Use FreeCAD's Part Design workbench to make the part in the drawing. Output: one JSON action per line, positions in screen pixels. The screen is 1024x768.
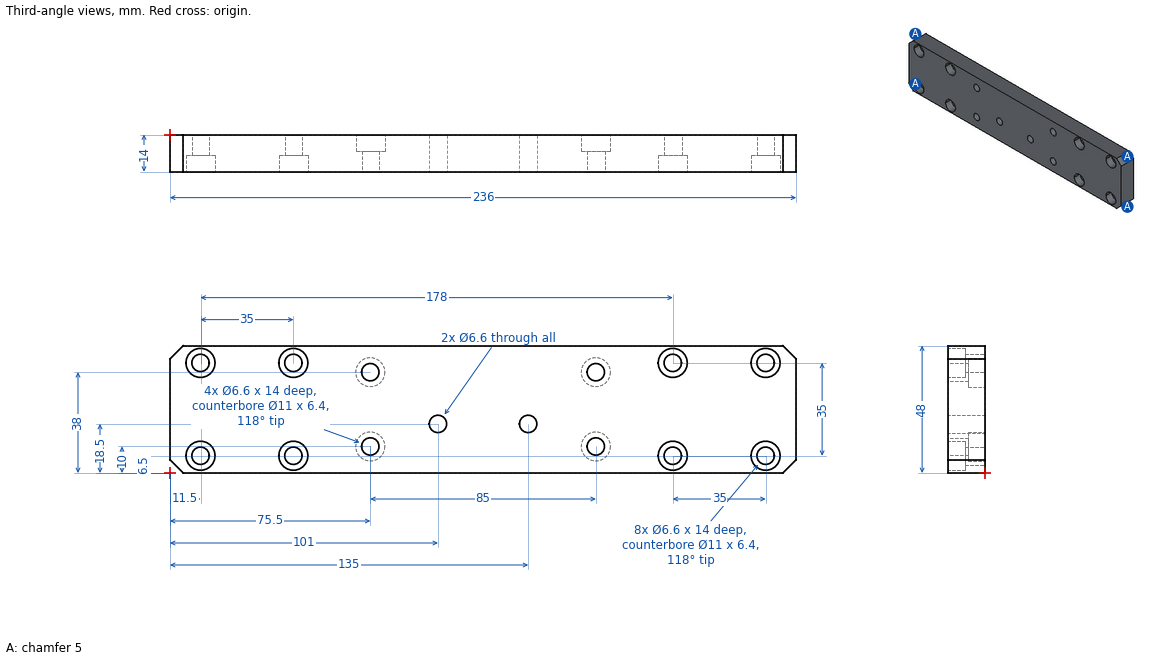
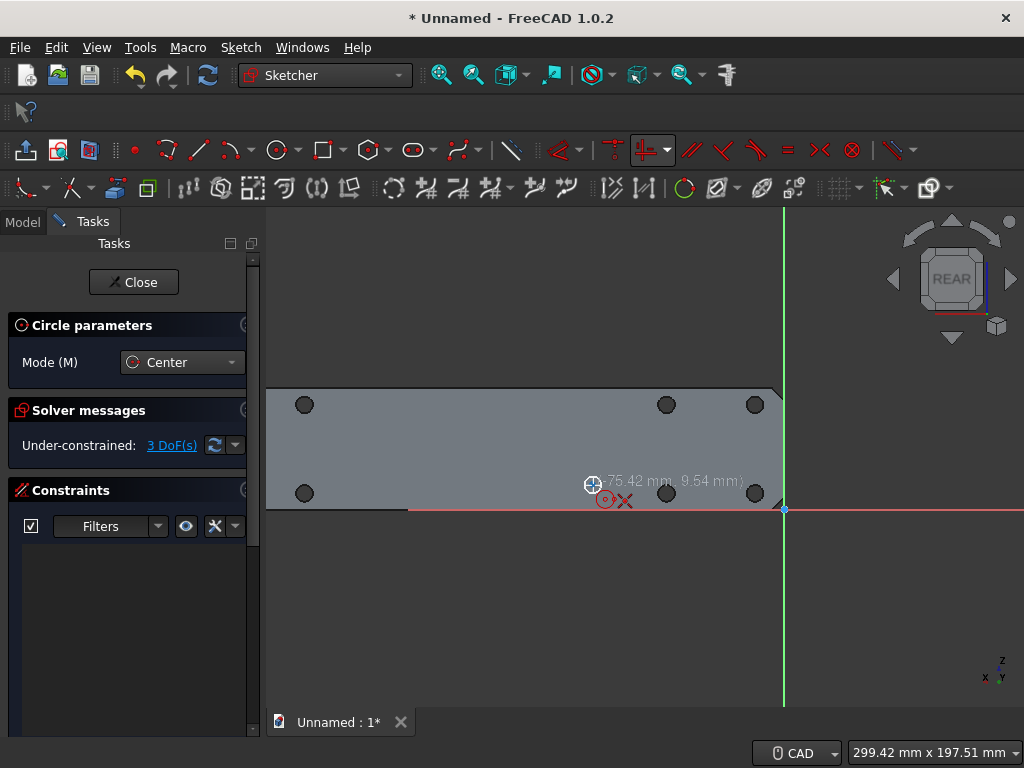
{"action": "scroll", "coordinate": [378, 485], "scroll_direction": "up", "scroll_amount": 5}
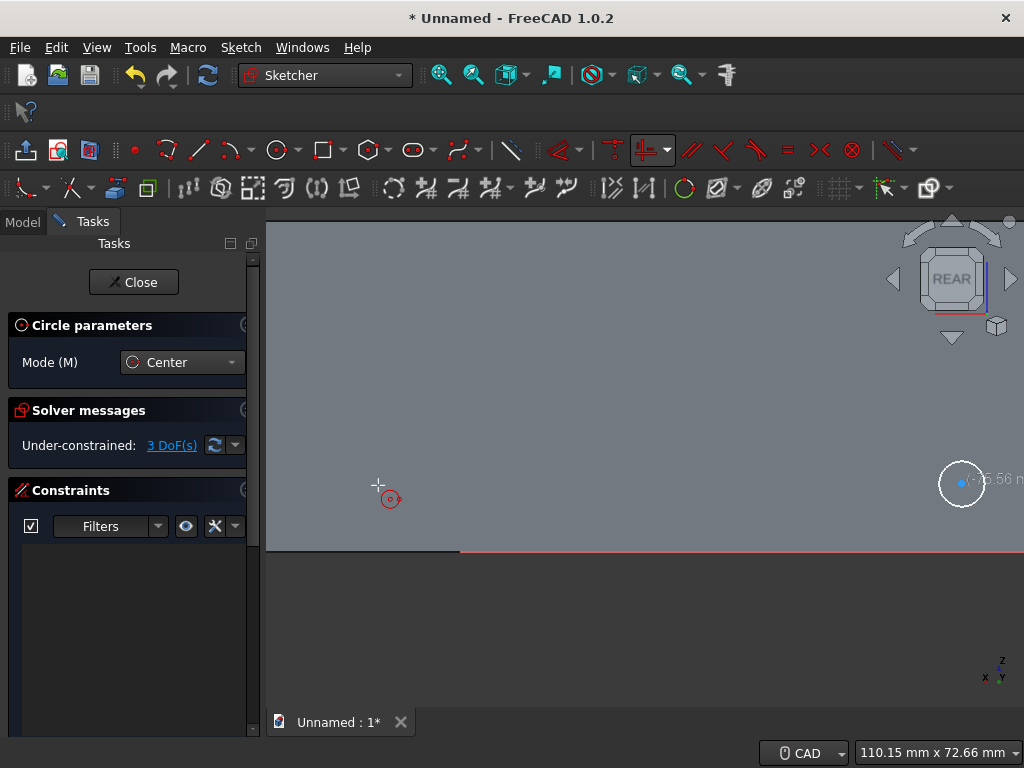
{"action": "left_click", "coordinate": [377, 483]}
{"action": "left_click", "coordinate": [393, 467]}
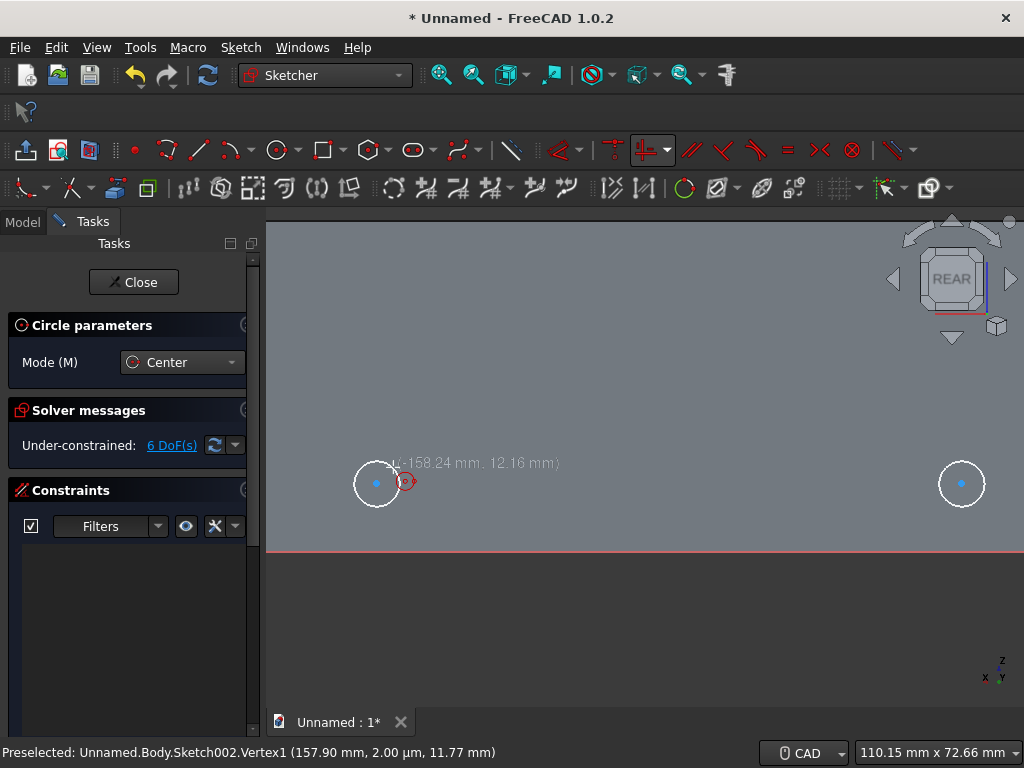
{"action": "scroll", "coordinate": [378, 485], "scroll_direction": "down", "scroll_amount": 5}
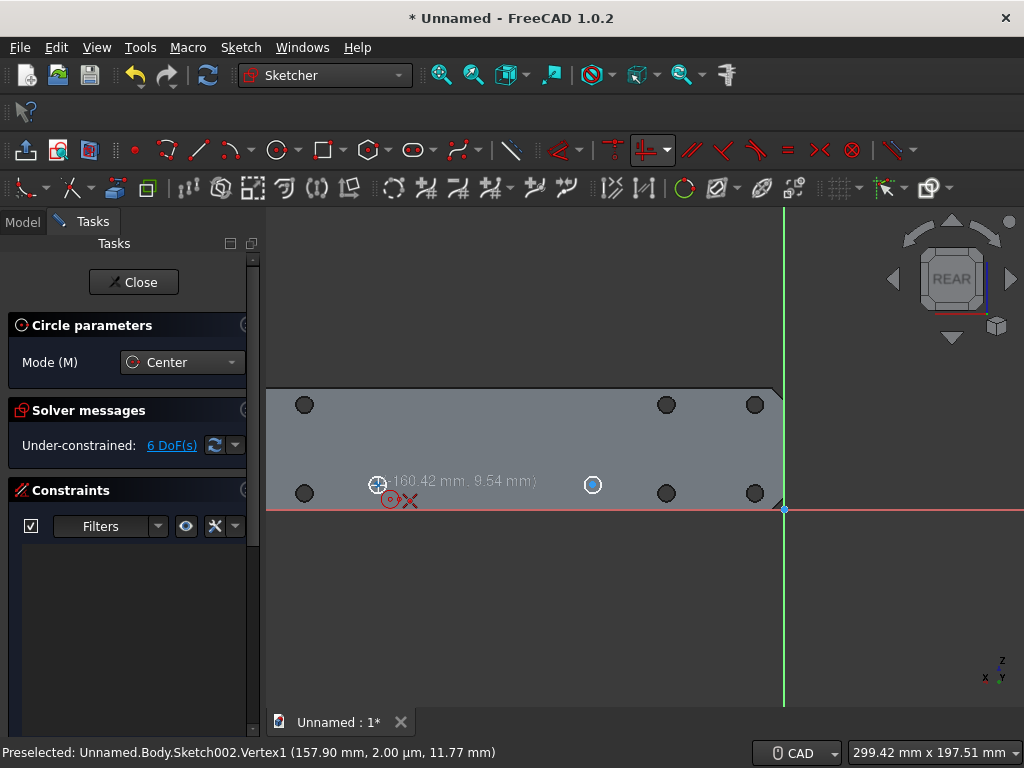
{"action": "scroll", "coordinate": [593, 414], "scroll_direction": "up", "scroll_amount": 5}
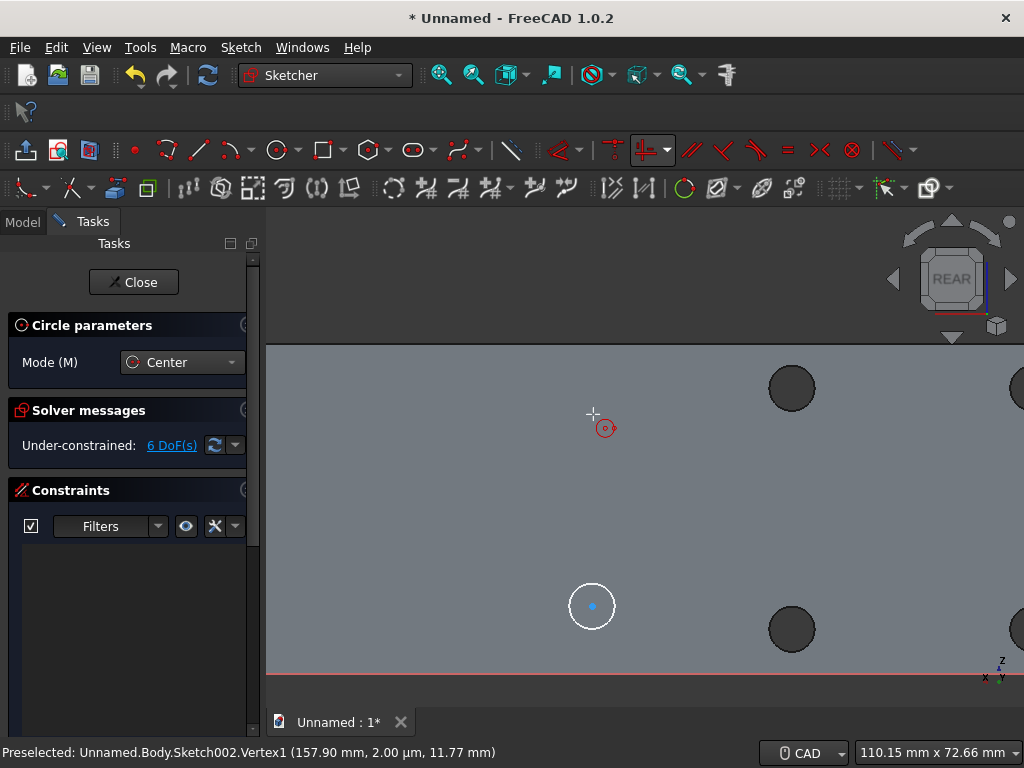
{"action": "left_click", "coordinate": [592, 412]}
{"action": "left_click", "coordinate": [608, 396]}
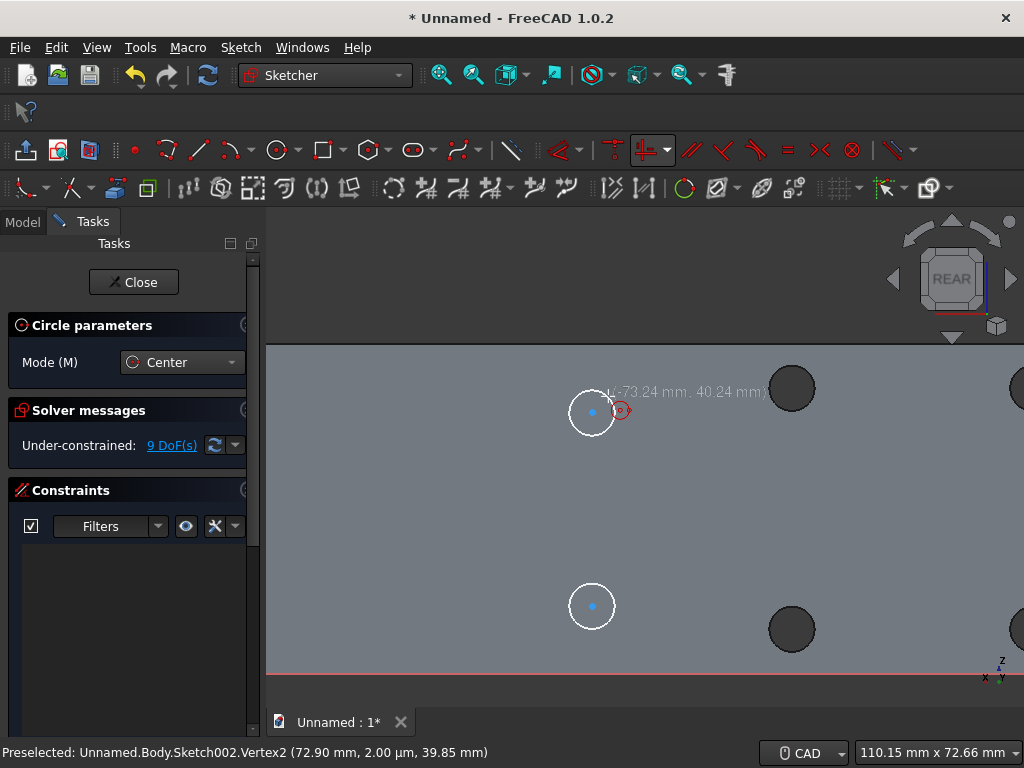
{"action": "scroll", "coordinate": [593, 413], "scroll_direction": "down", "scroll_amount": 5}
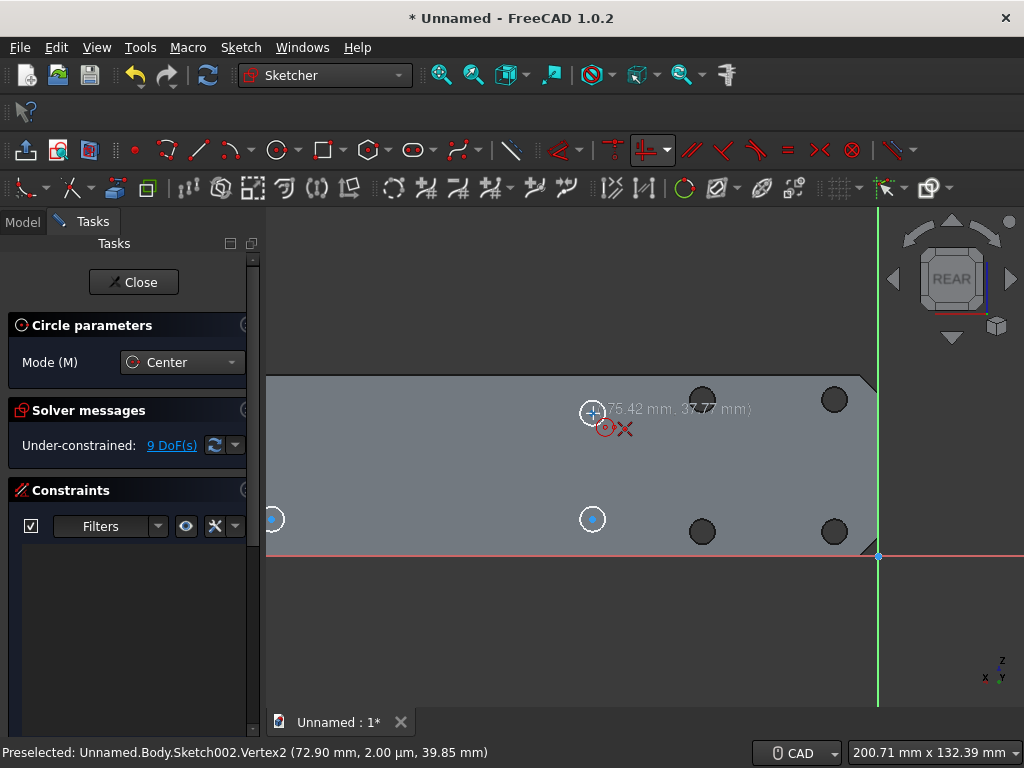
{"action": "scroll", "coordinate": [378, 413], "scroll_direction": "up", "scroll_amount": 5}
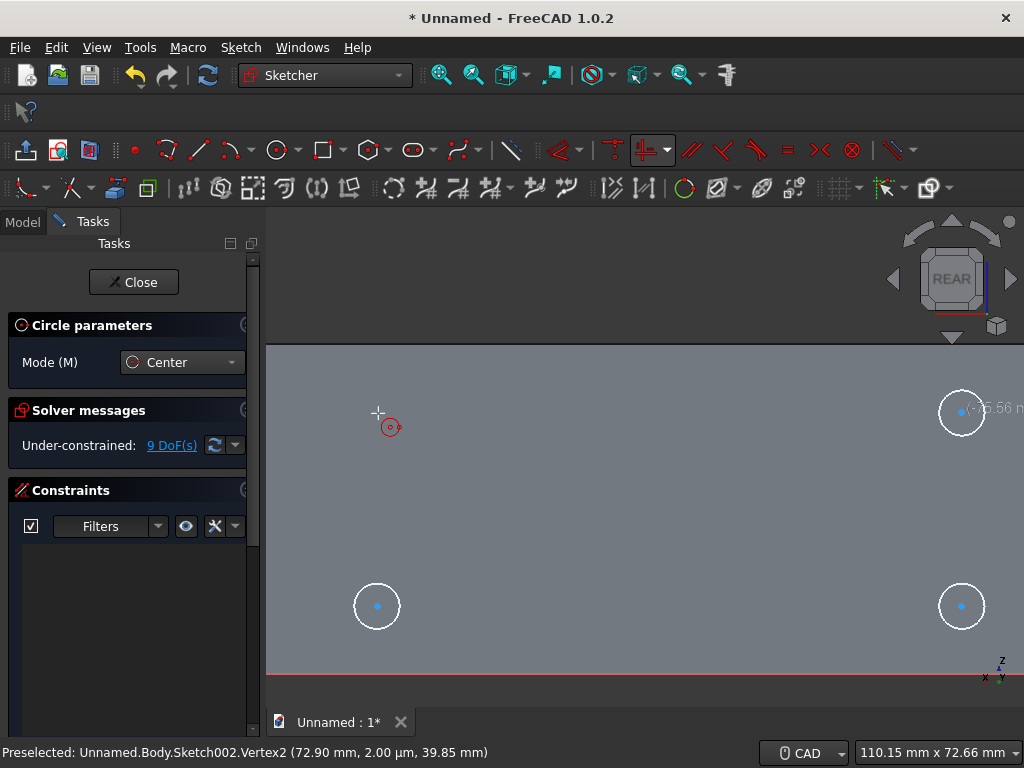
{"action": "left_click", "coordinate": [377, 412]}
{"action": "left_click", "coordinate": [393, 396]}
{"action": "key", "text": "Escape"}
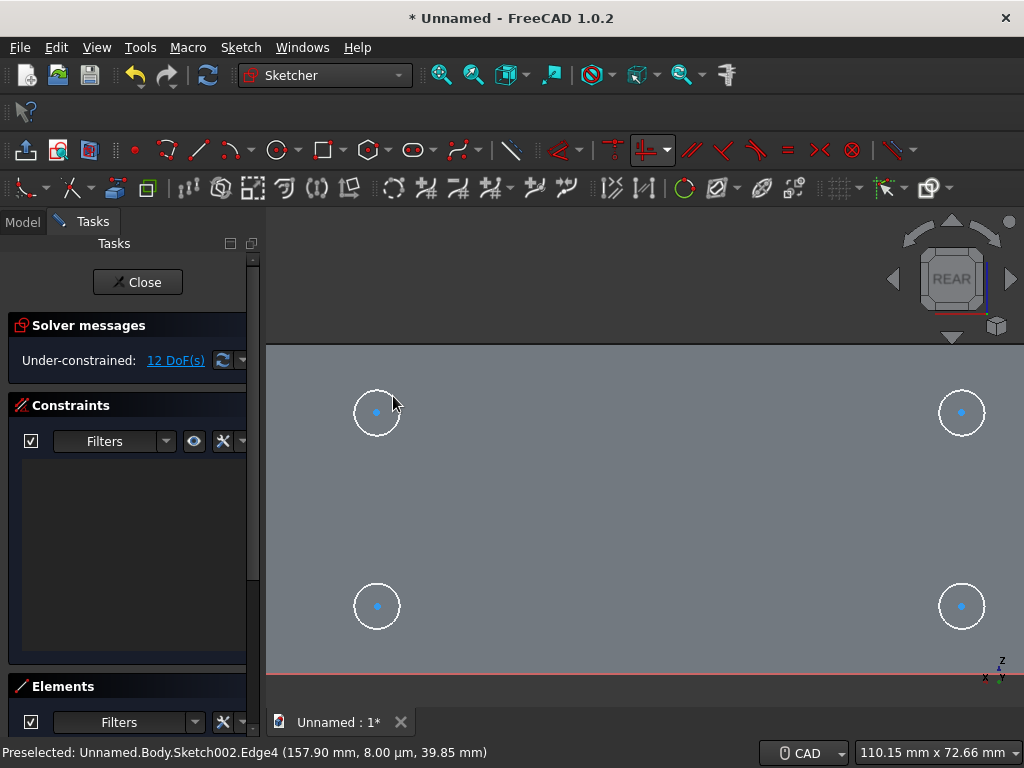
{"action": "scroll", "coordinate": [378, 413], "scroll_direction": "down", "scroll_amount": 5}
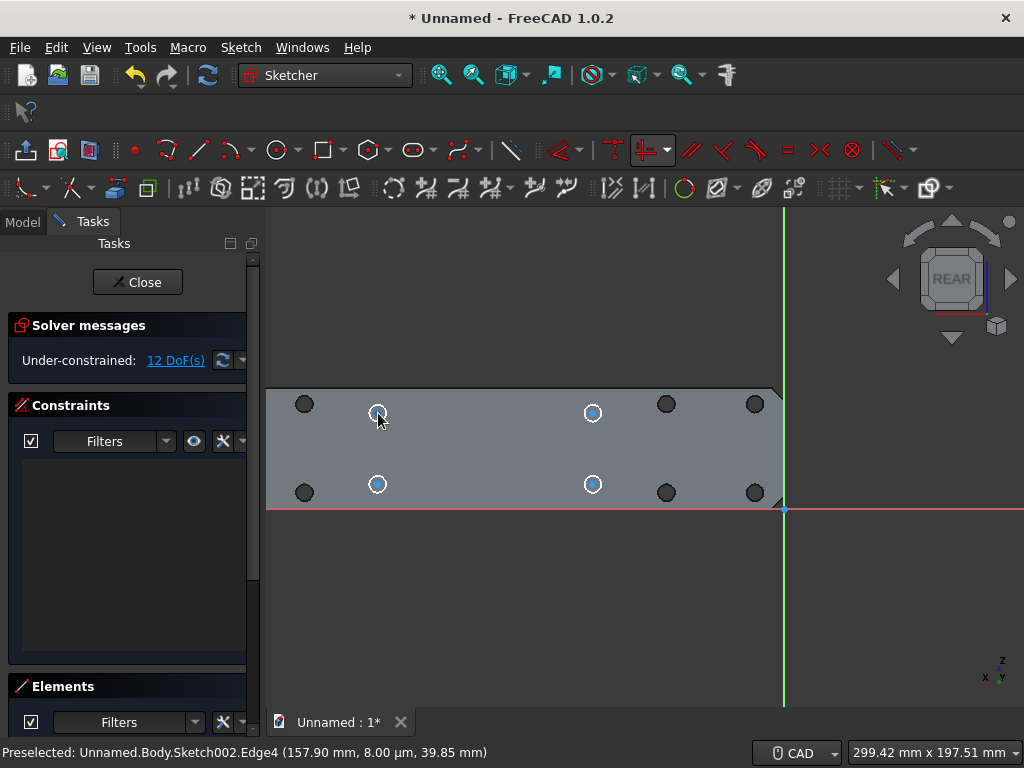
{"action": "scroll", "coordinate": [599, 478], "scroll_direction": "up", "scroll_amount": 3}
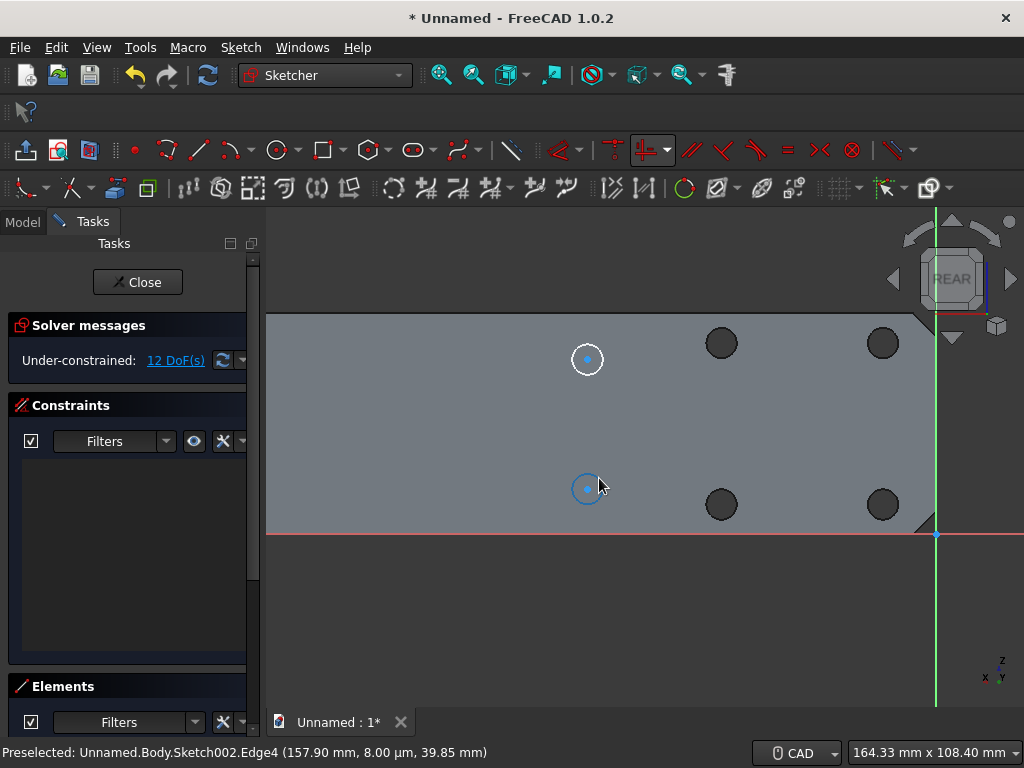
{"action": "left_click", "coordinate": [598, 478]}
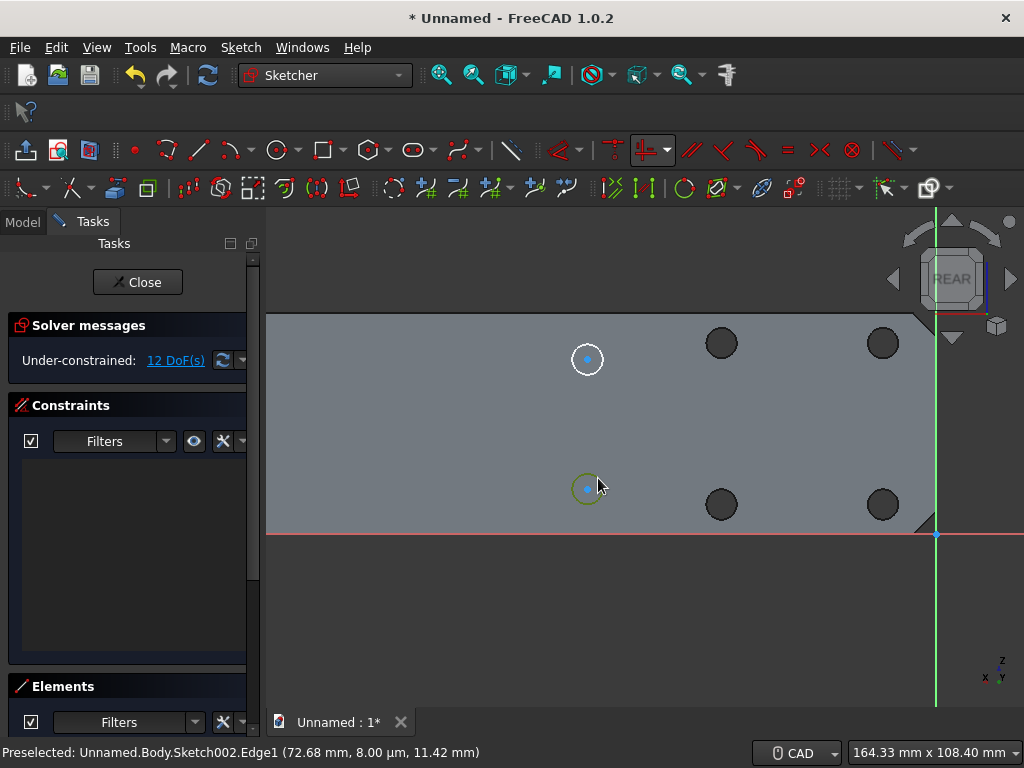
{"action": "scroll", "coordinate": [599, 479], "scroll_direction": "down", "scroll_amount": 3}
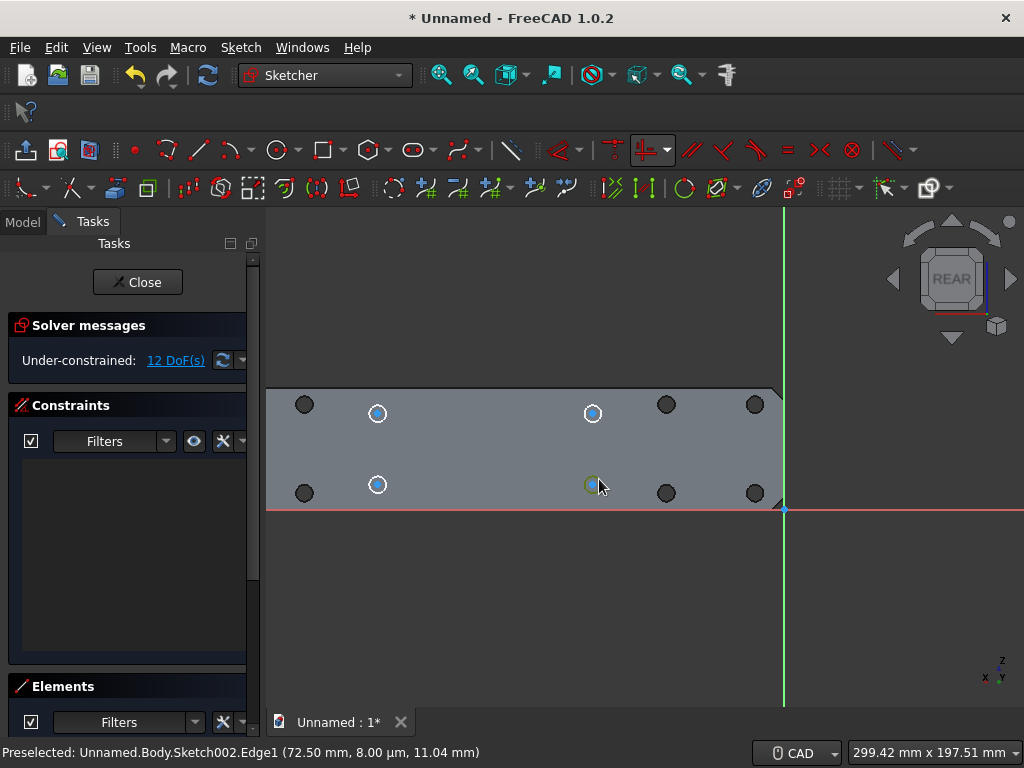
{"action": "scroll", "coordinate": [384, 479], "scroll_direction": "up", "scroll_amount": 3}